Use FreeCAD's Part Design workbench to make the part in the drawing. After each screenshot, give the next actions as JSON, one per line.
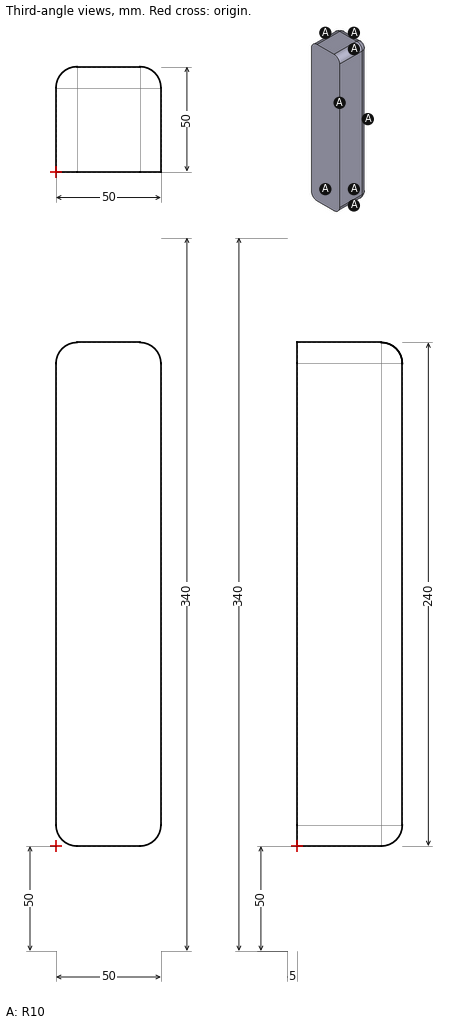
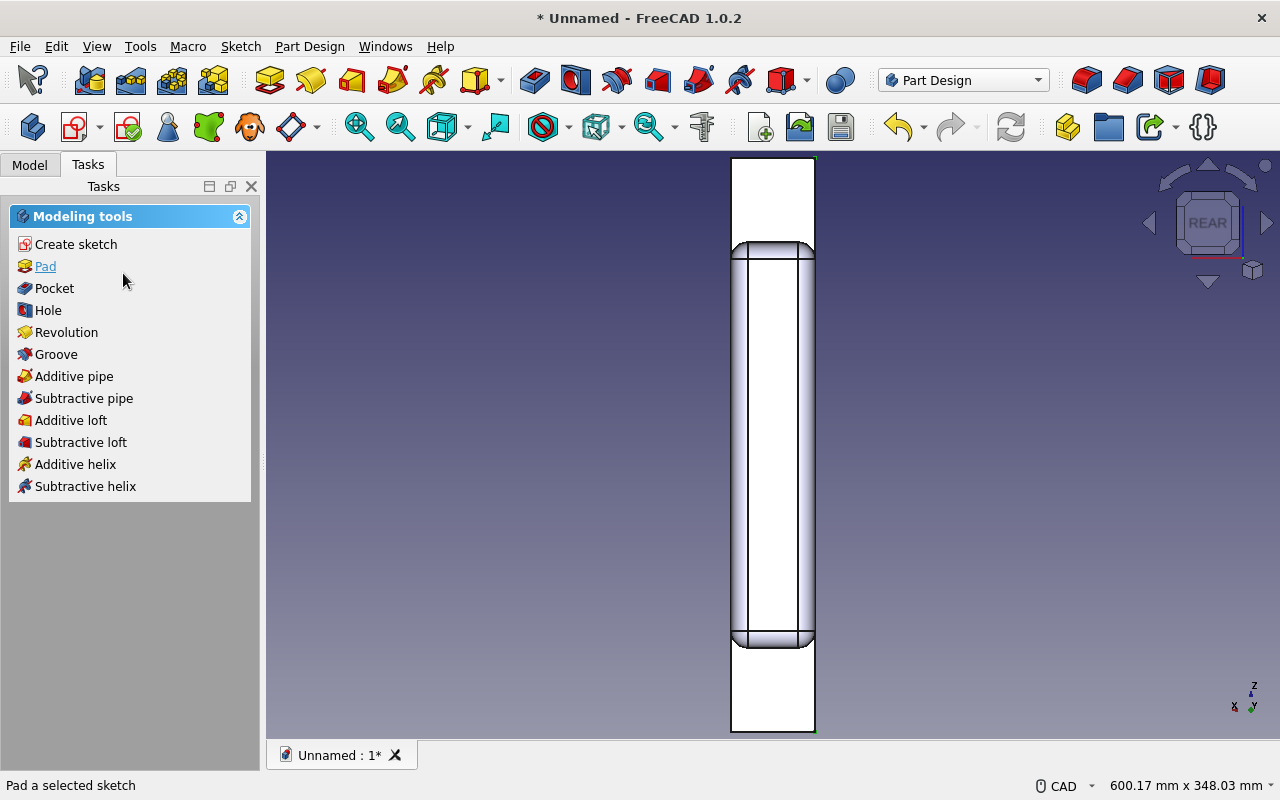
{"action": "left_click", "coordinate": [535, 80]}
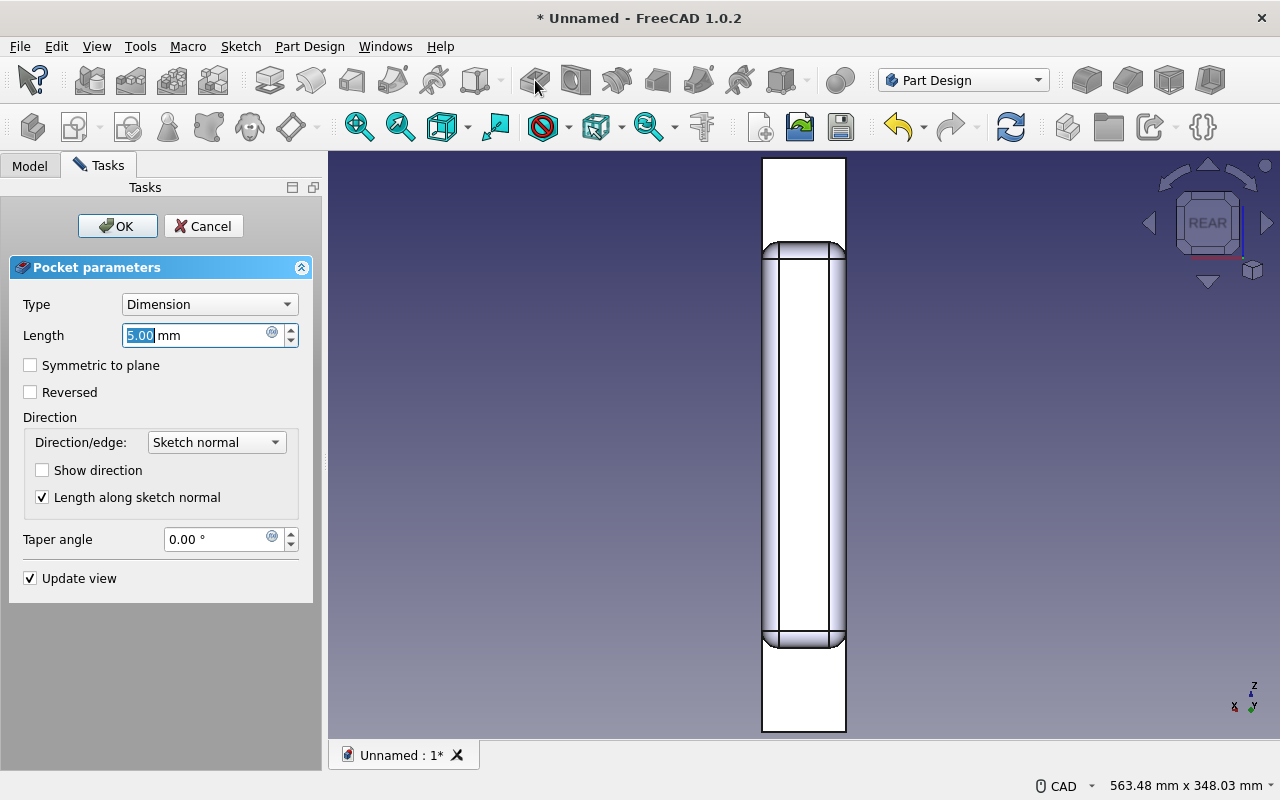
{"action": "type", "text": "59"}
{"action": "key", "text": "Tab"}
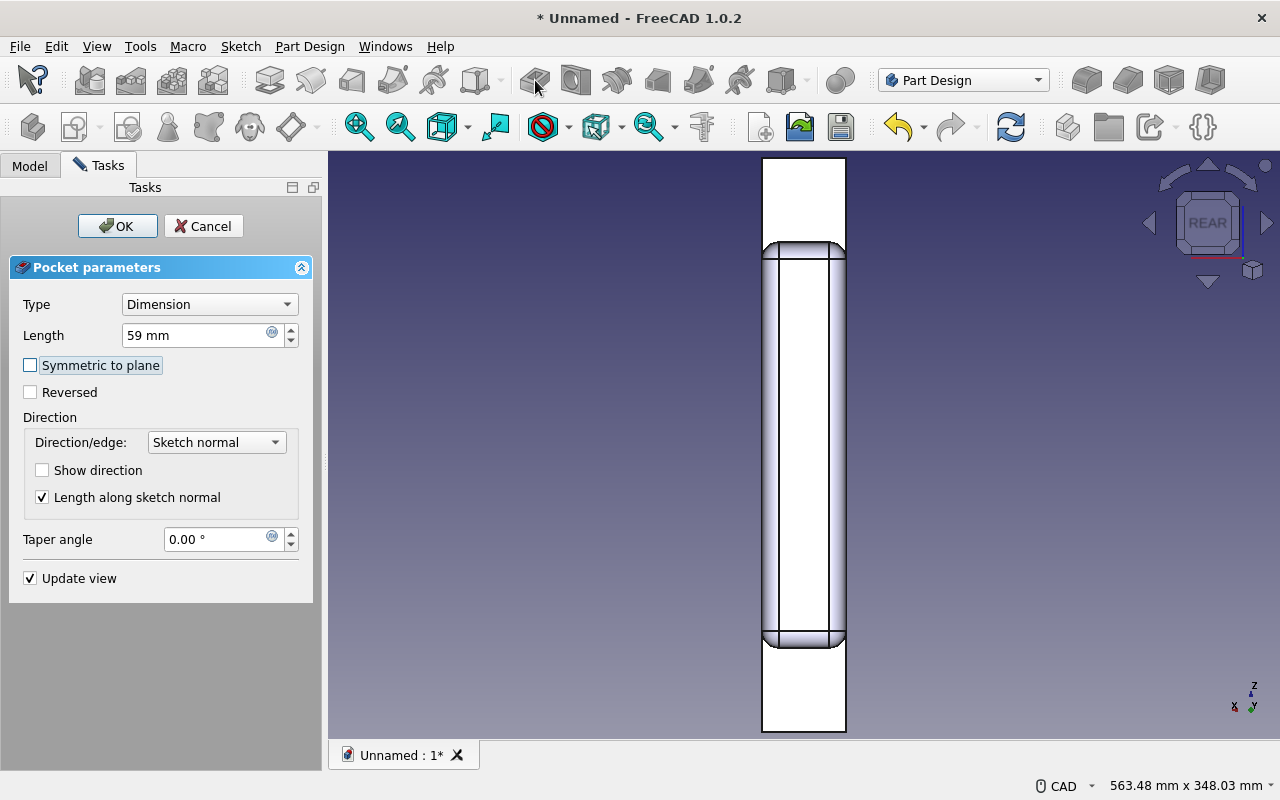
{"action": "left_click", "coordinate": [31, 392]}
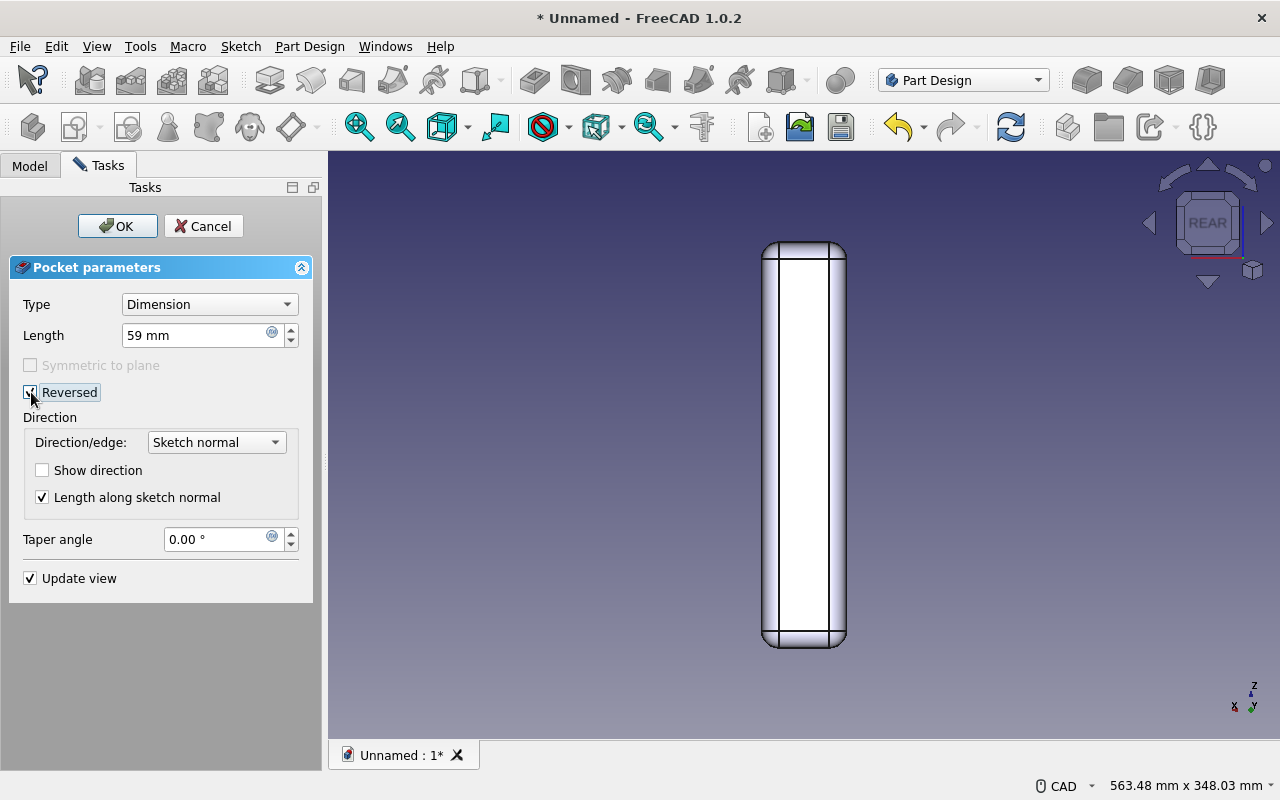
{"action": "left_click", "coordinate": [118, 226]}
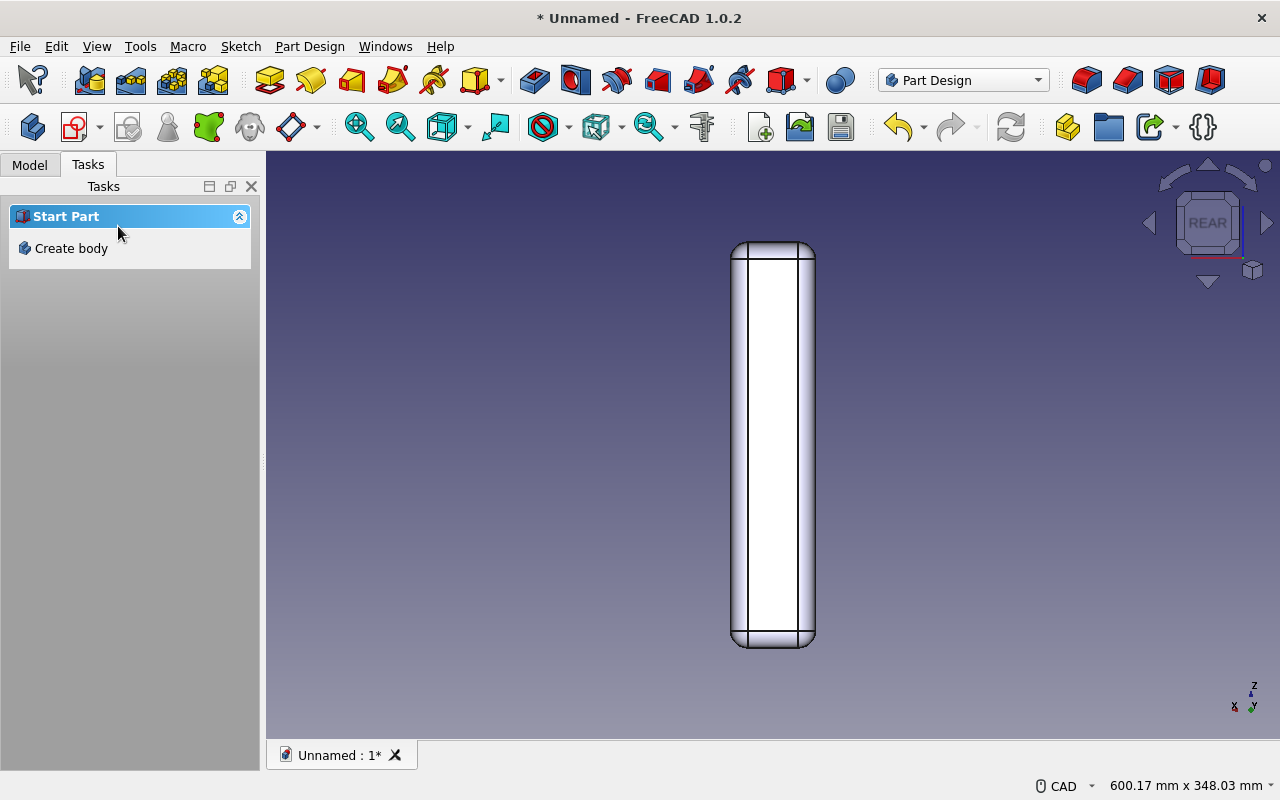
{"action": "key", "text": "0"}